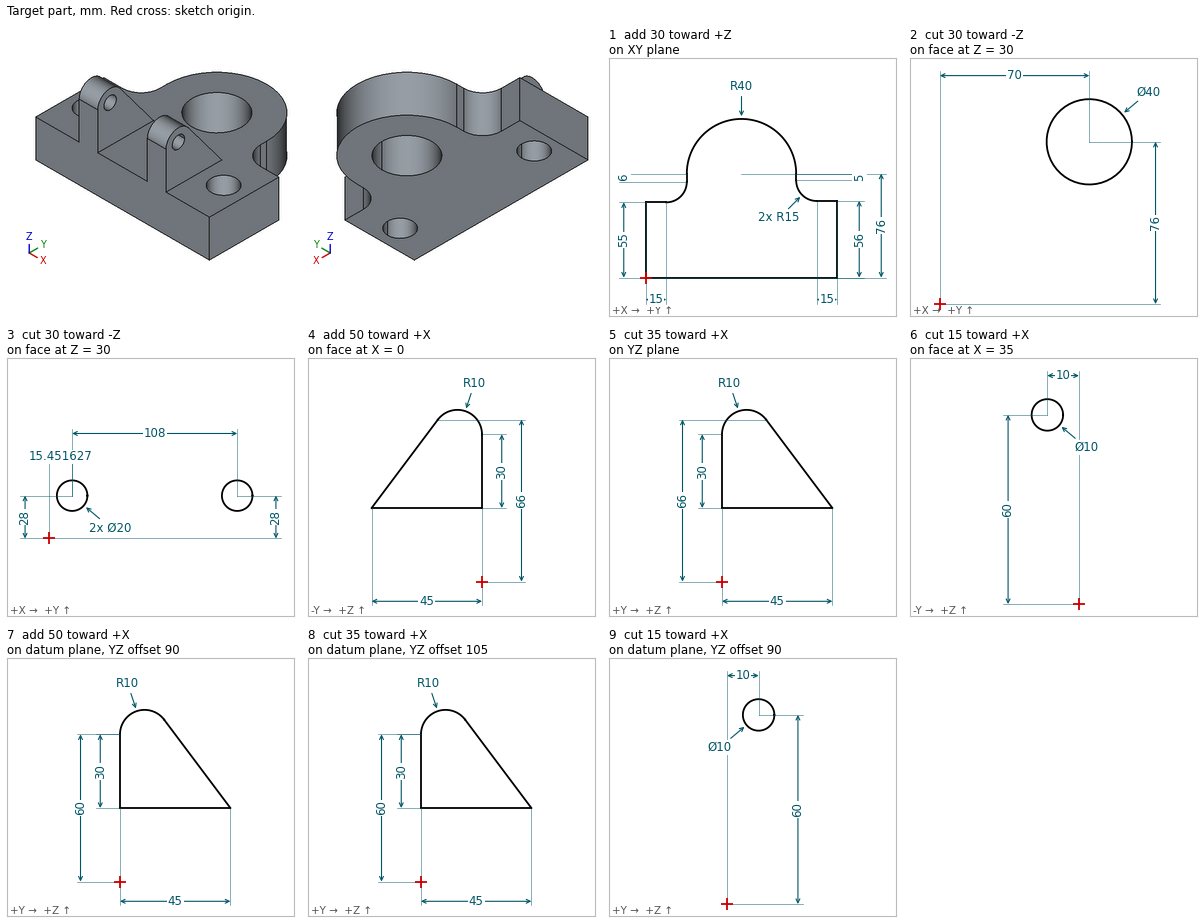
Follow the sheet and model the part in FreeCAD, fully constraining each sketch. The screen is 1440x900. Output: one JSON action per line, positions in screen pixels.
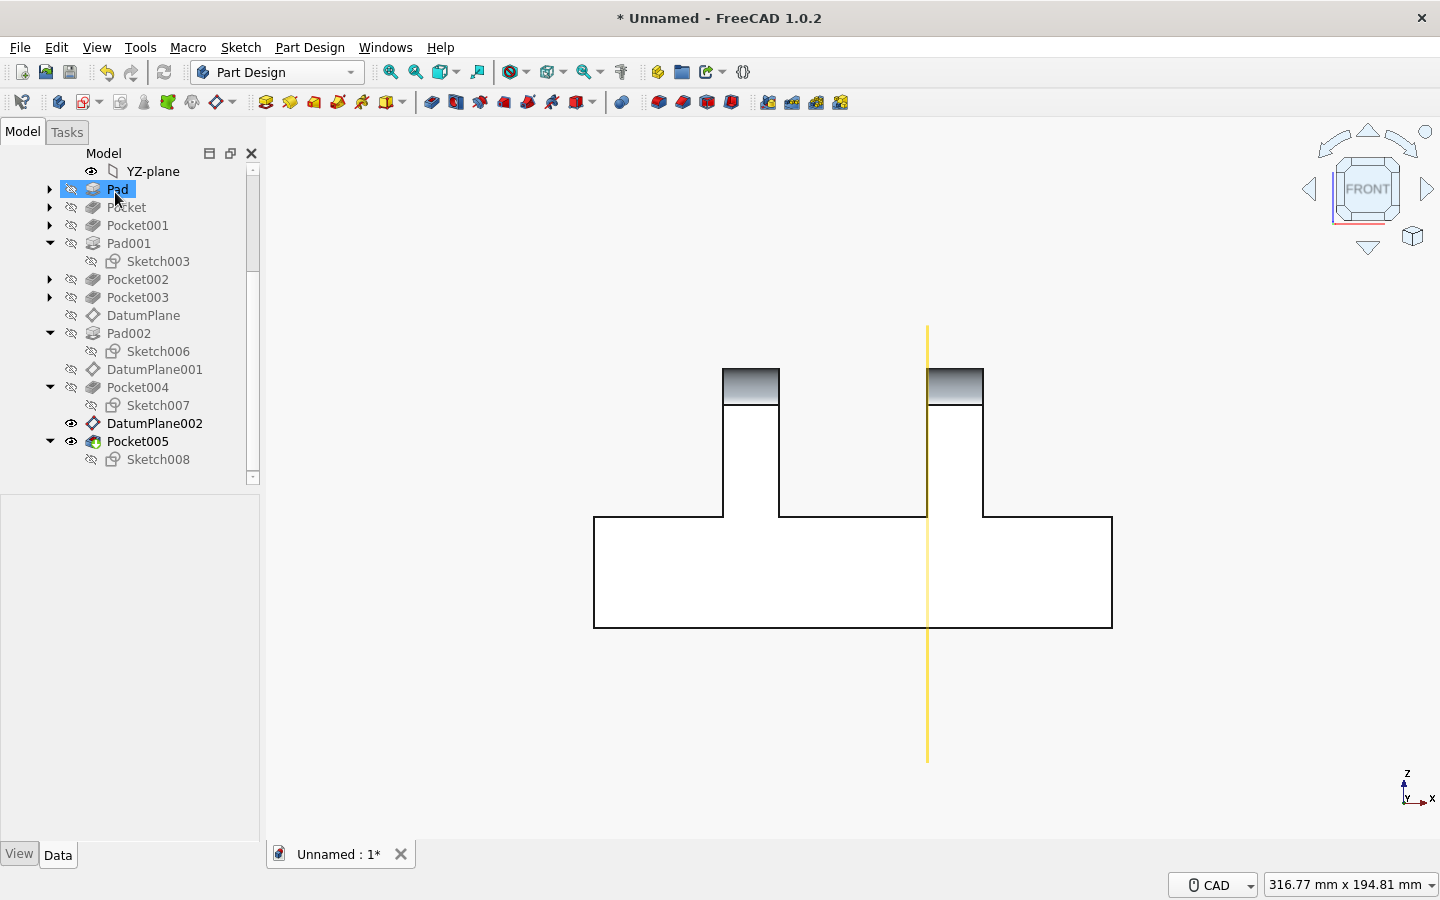
{"action": "left_click", "coordinate": [116, 423]}
{"action": "key", "text": "space"}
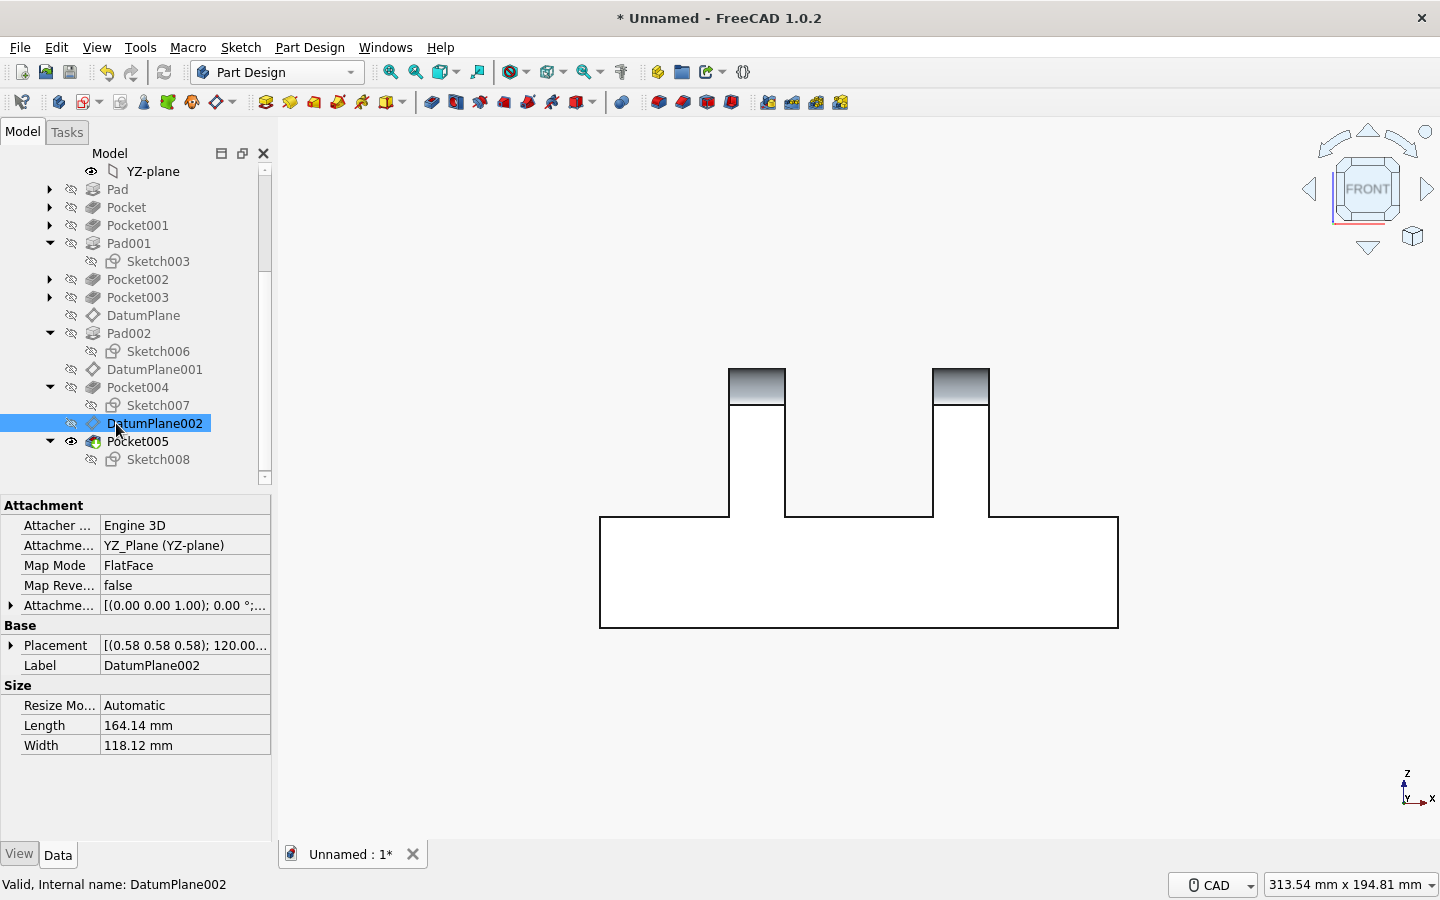
{"action": "key", "text": "0"}